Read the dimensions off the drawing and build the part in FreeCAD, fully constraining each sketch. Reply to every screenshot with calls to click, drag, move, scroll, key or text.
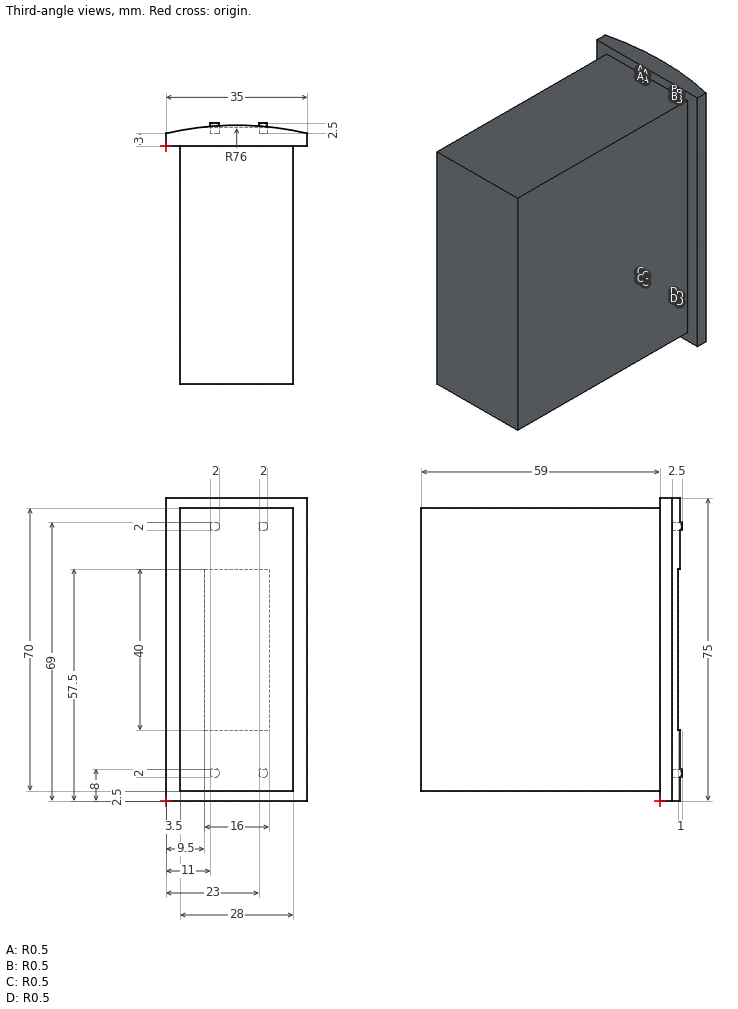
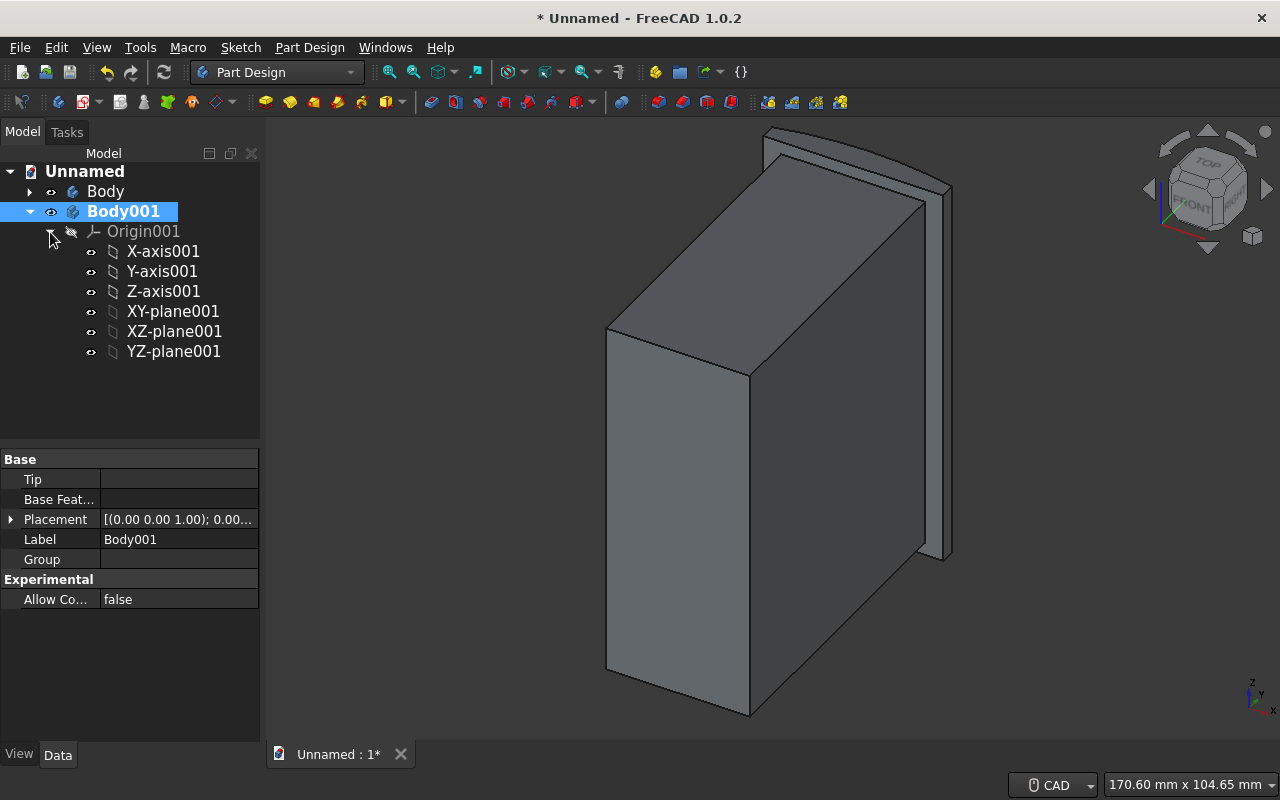
click(136, 332)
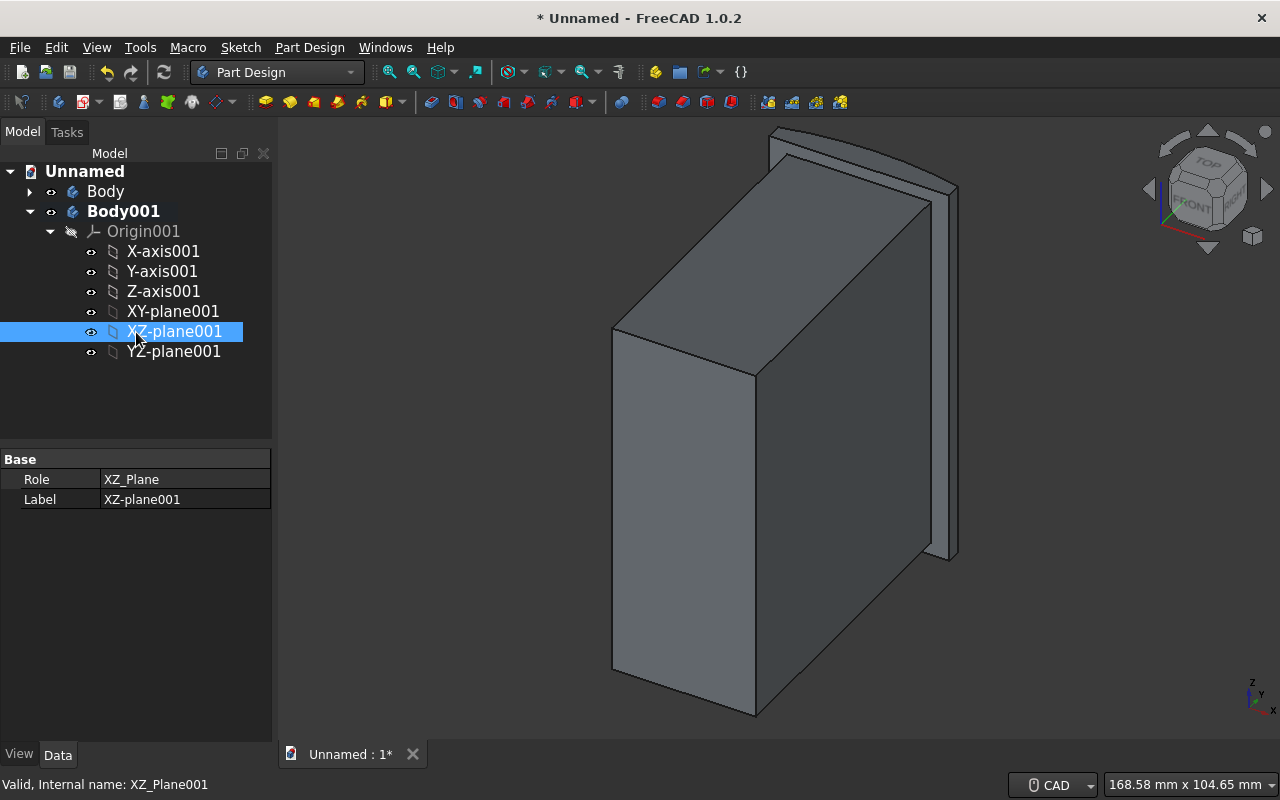
click(216, 102)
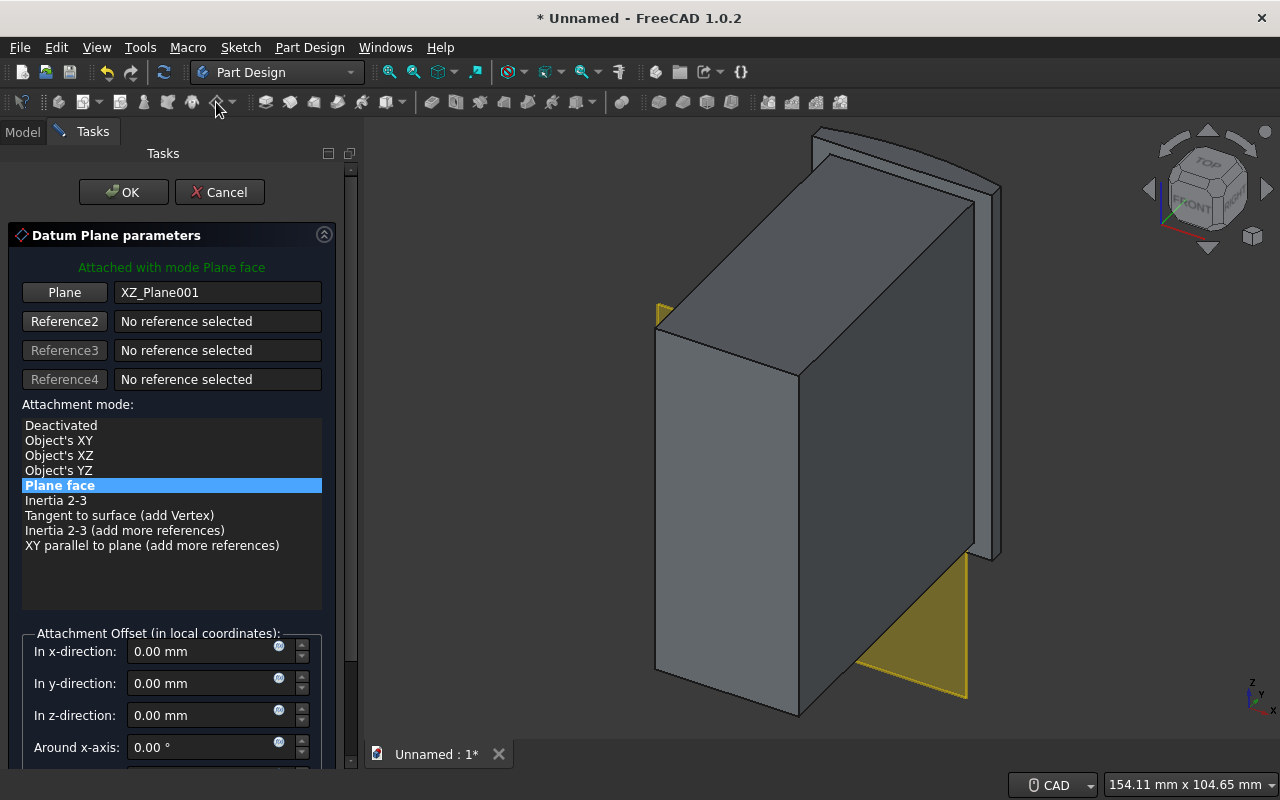
triple_click(210, 715)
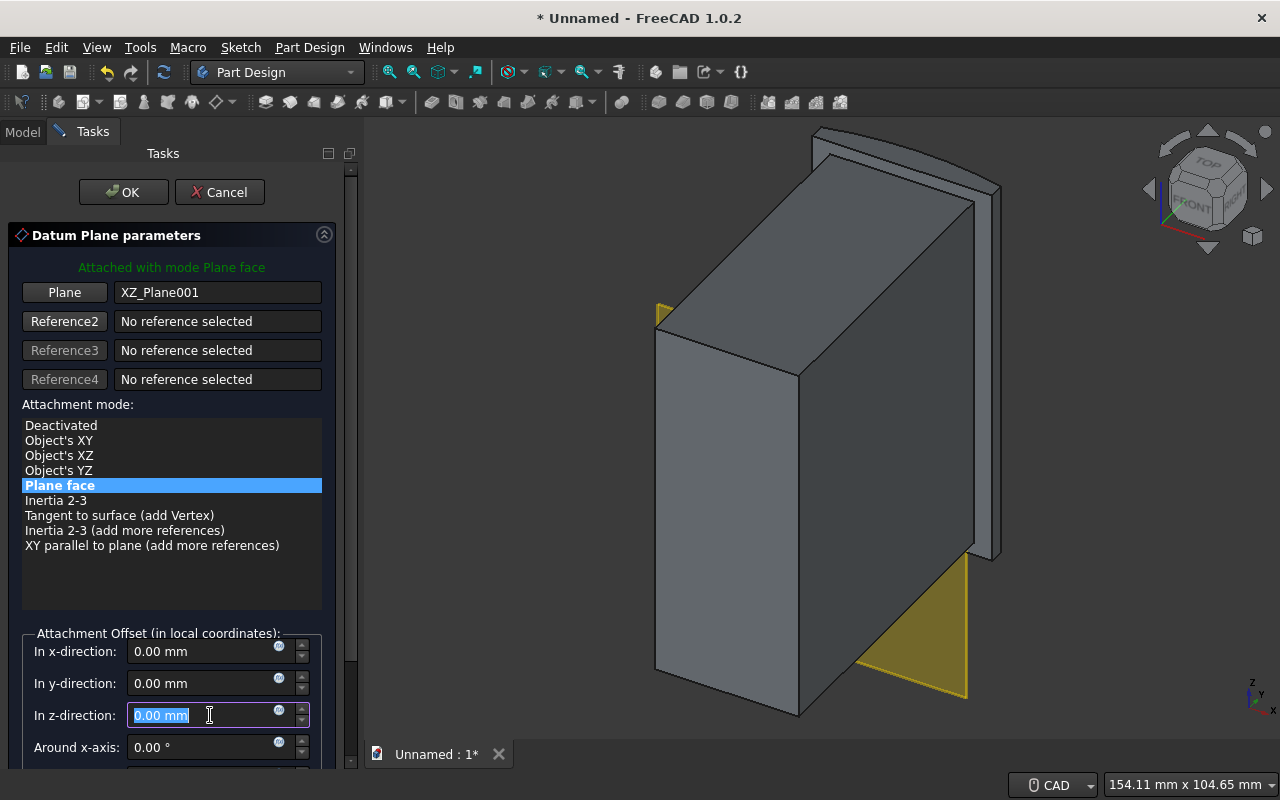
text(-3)
key(Tab)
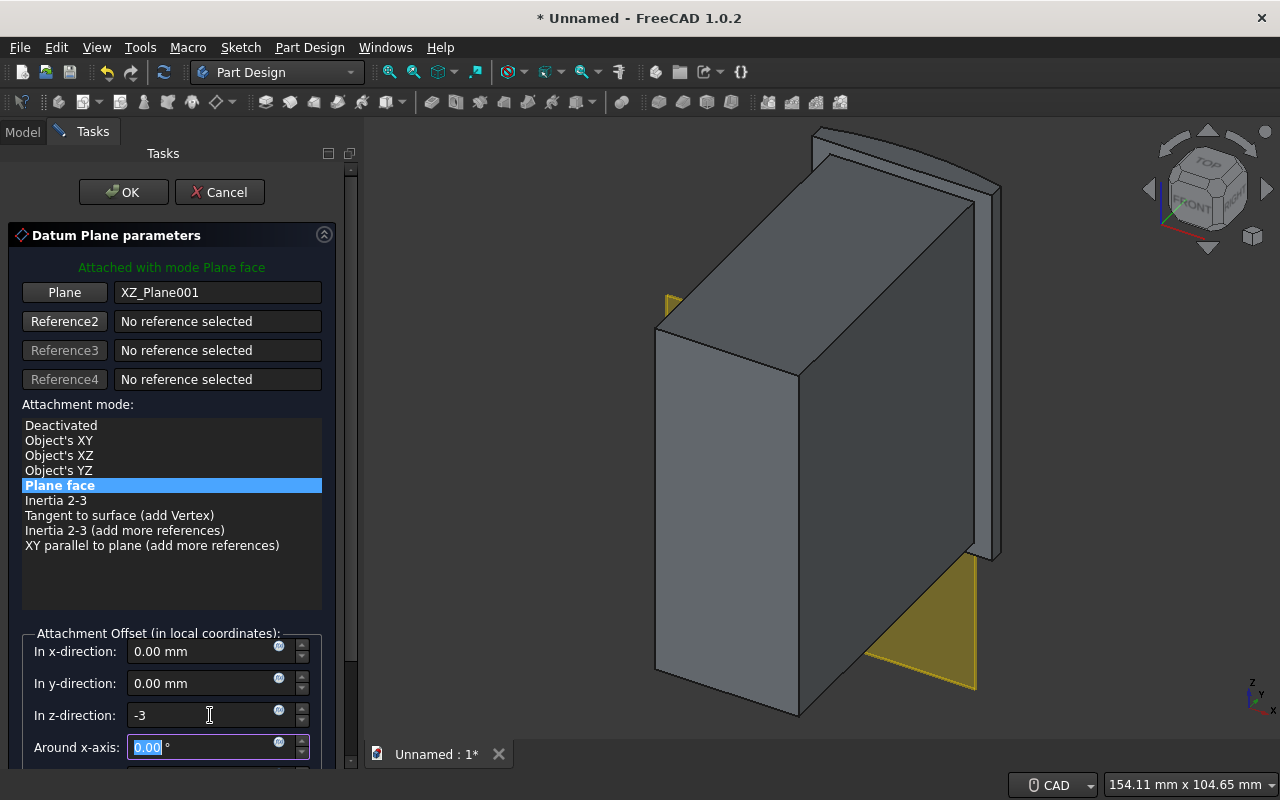
click(124, 192)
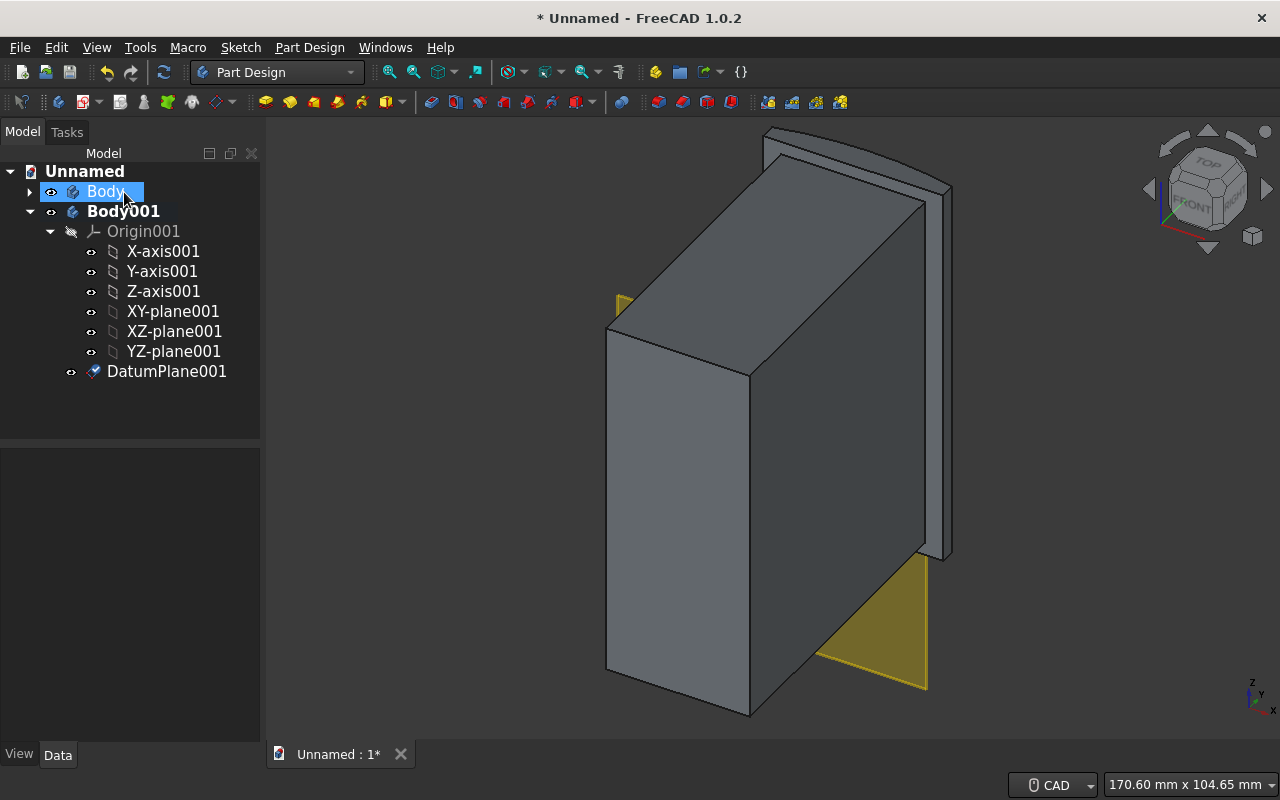
click(116, 372)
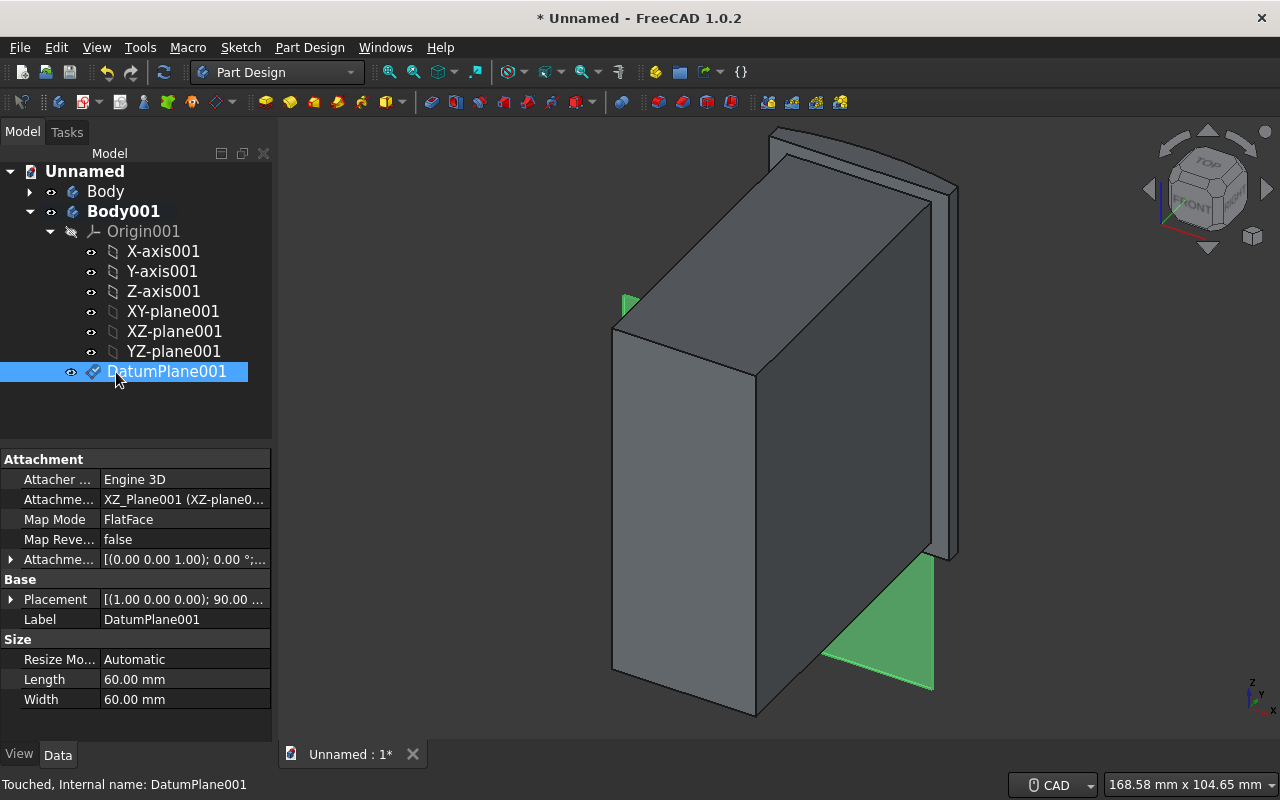
click(84, 102)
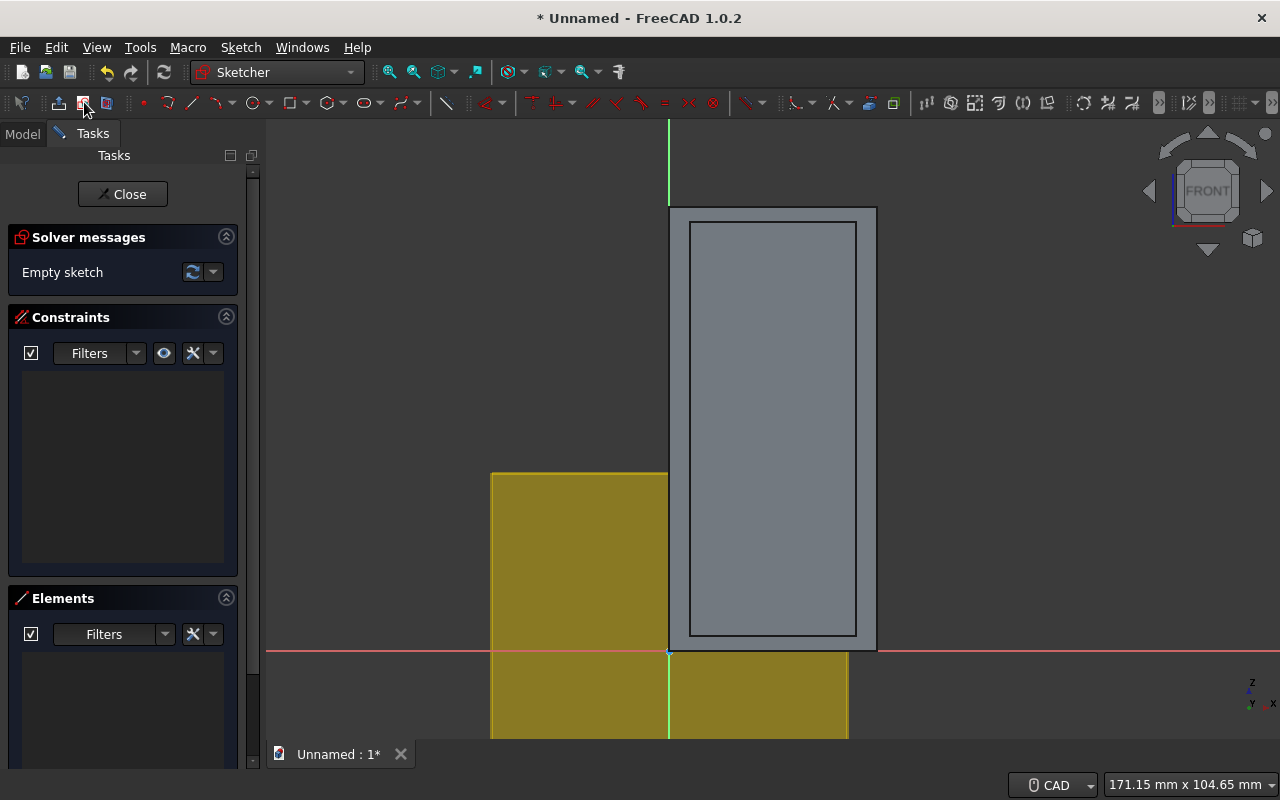
scroll(742, 239, up, 15)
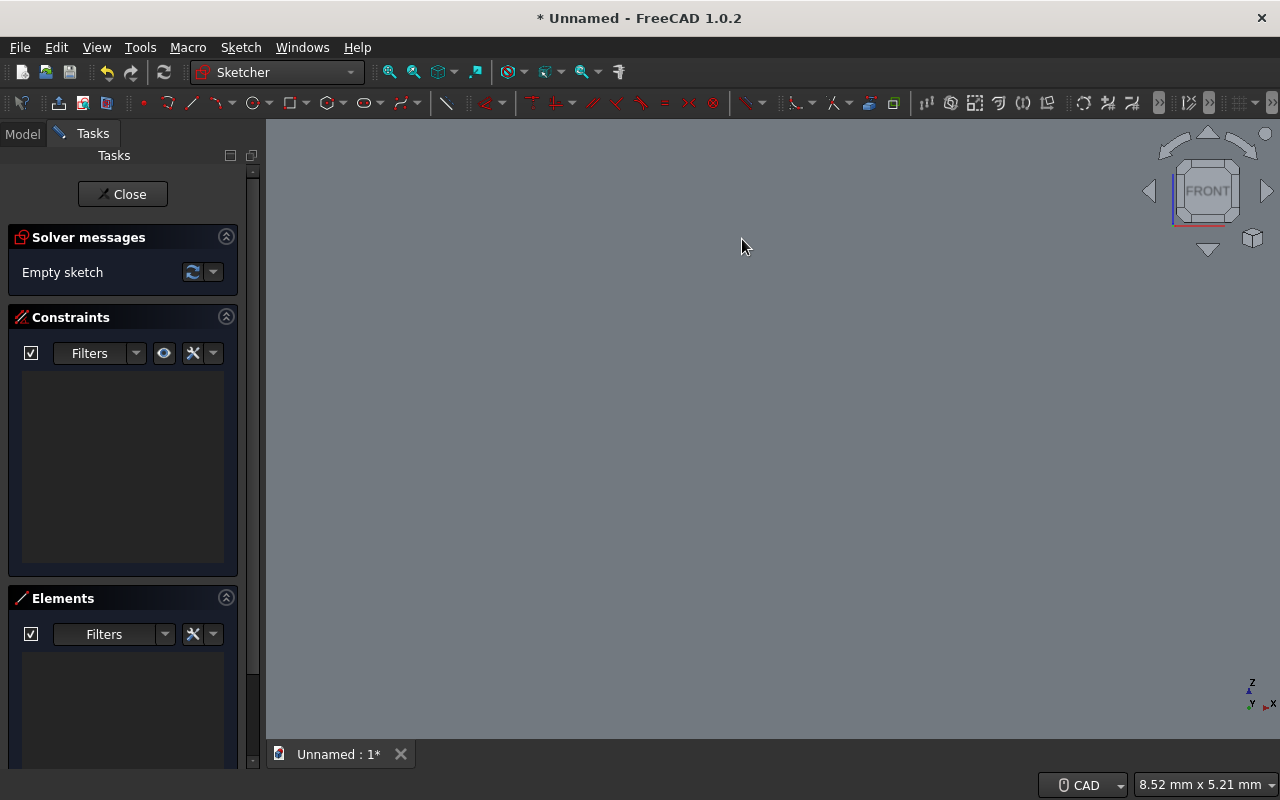
scroll(697, 414, up, 3)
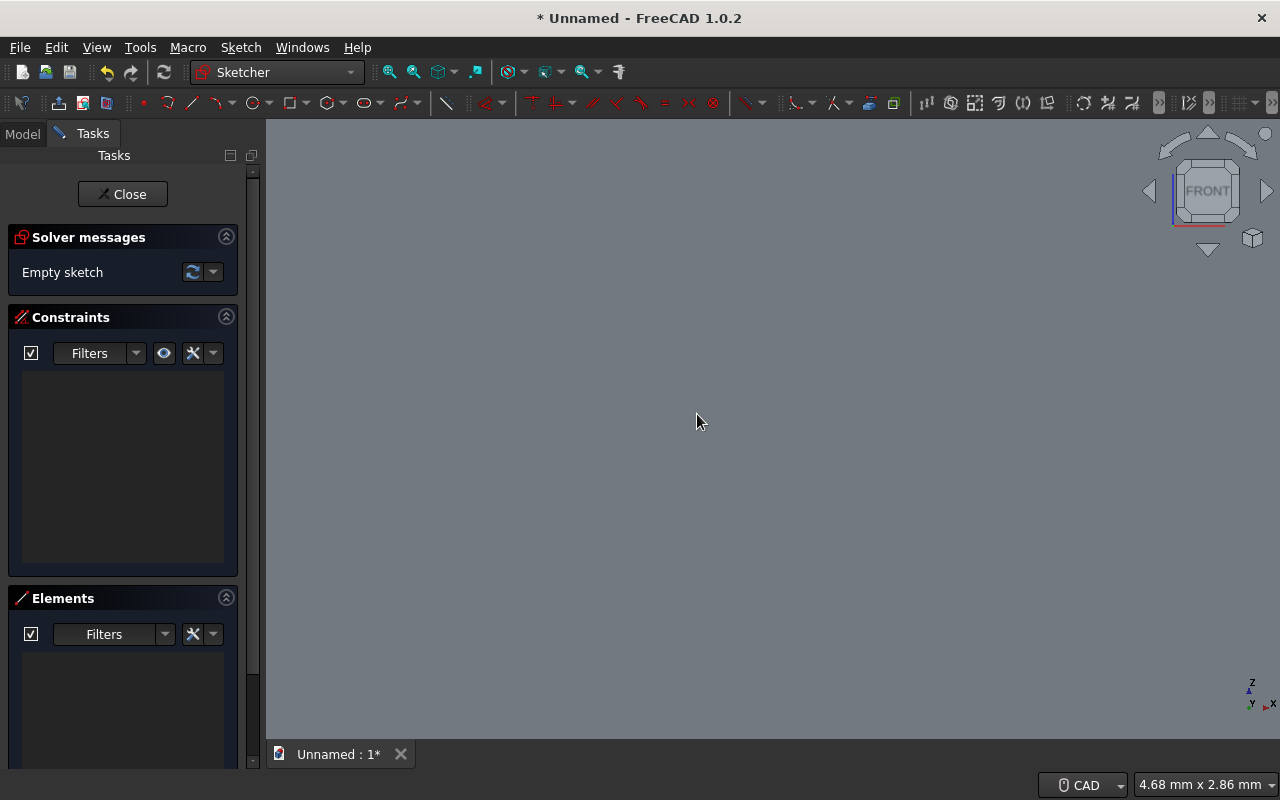
key(g)
key(r)